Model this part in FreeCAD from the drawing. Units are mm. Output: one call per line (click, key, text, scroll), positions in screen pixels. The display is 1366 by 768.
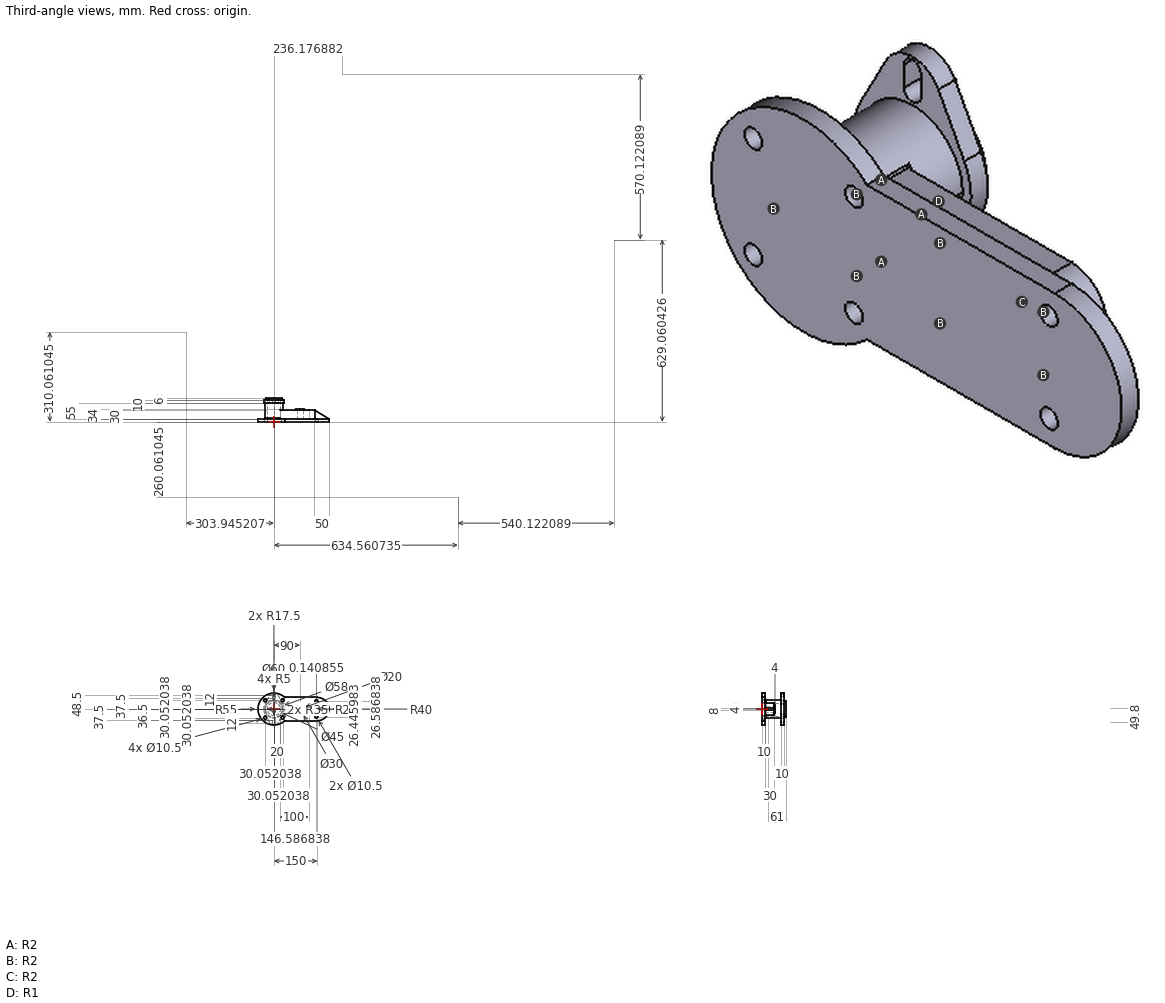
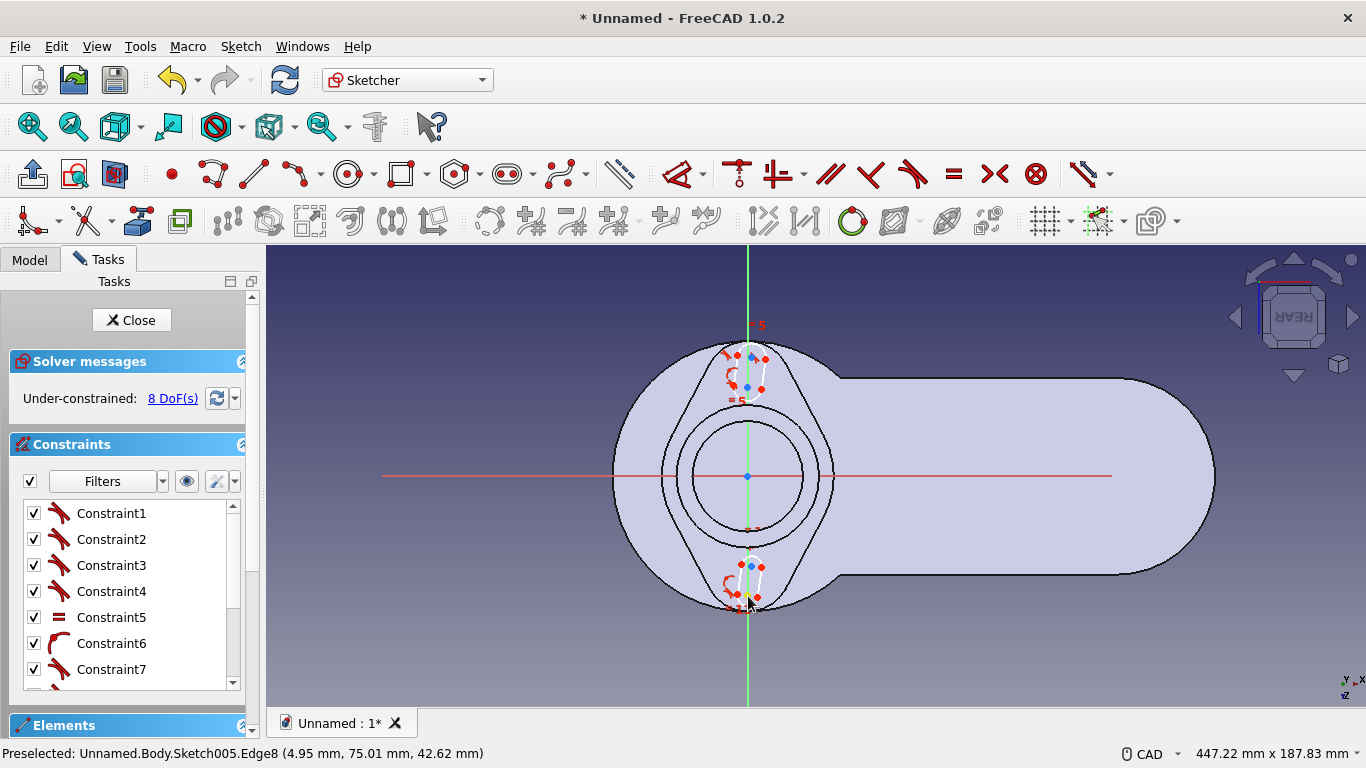
scroll(735, 376, up, 3)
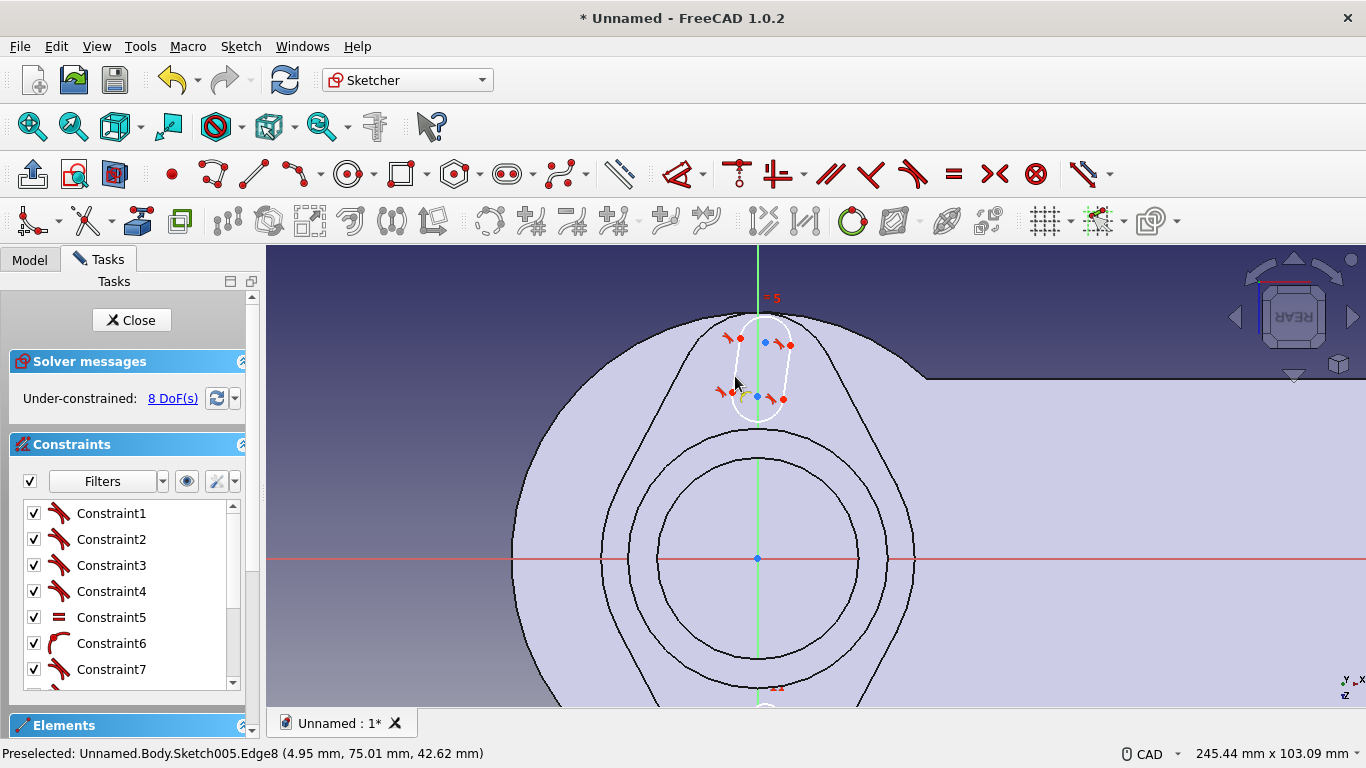
click(735, 376)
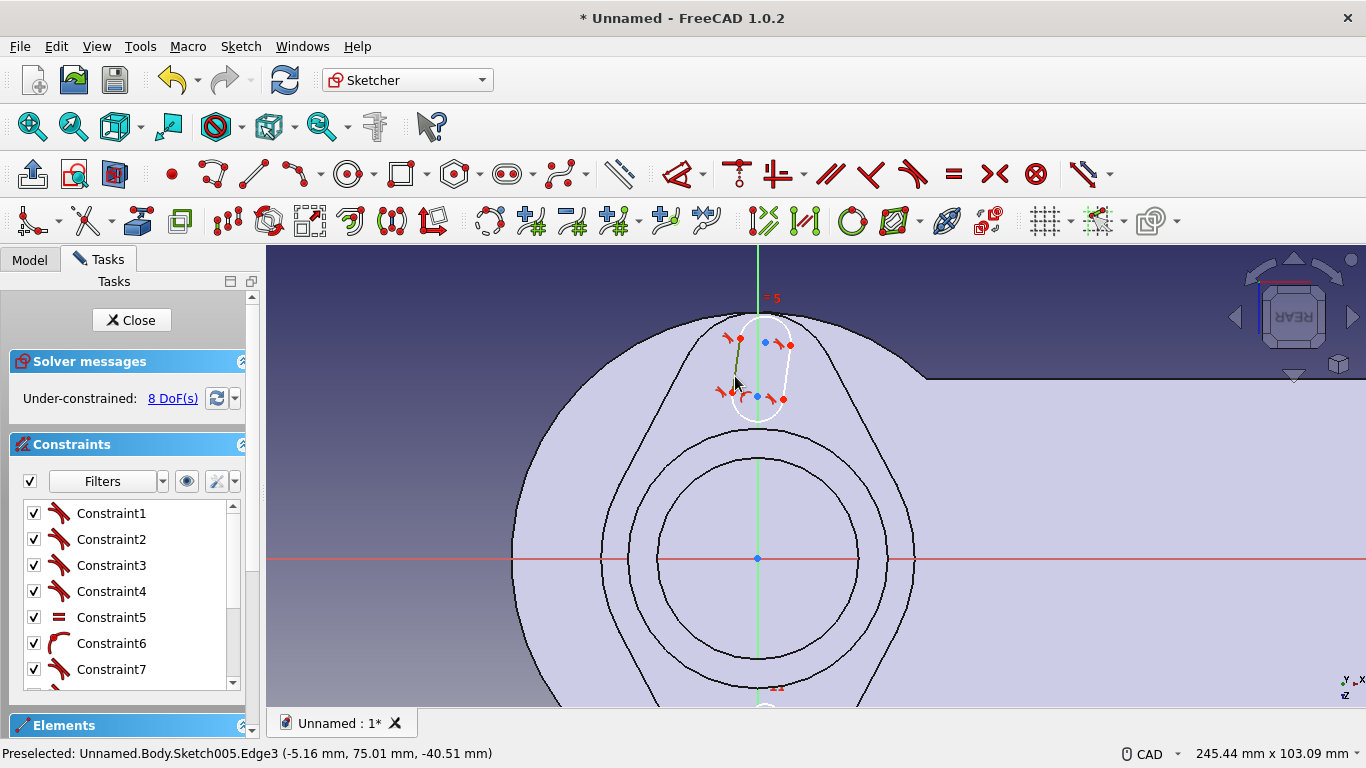
key(v)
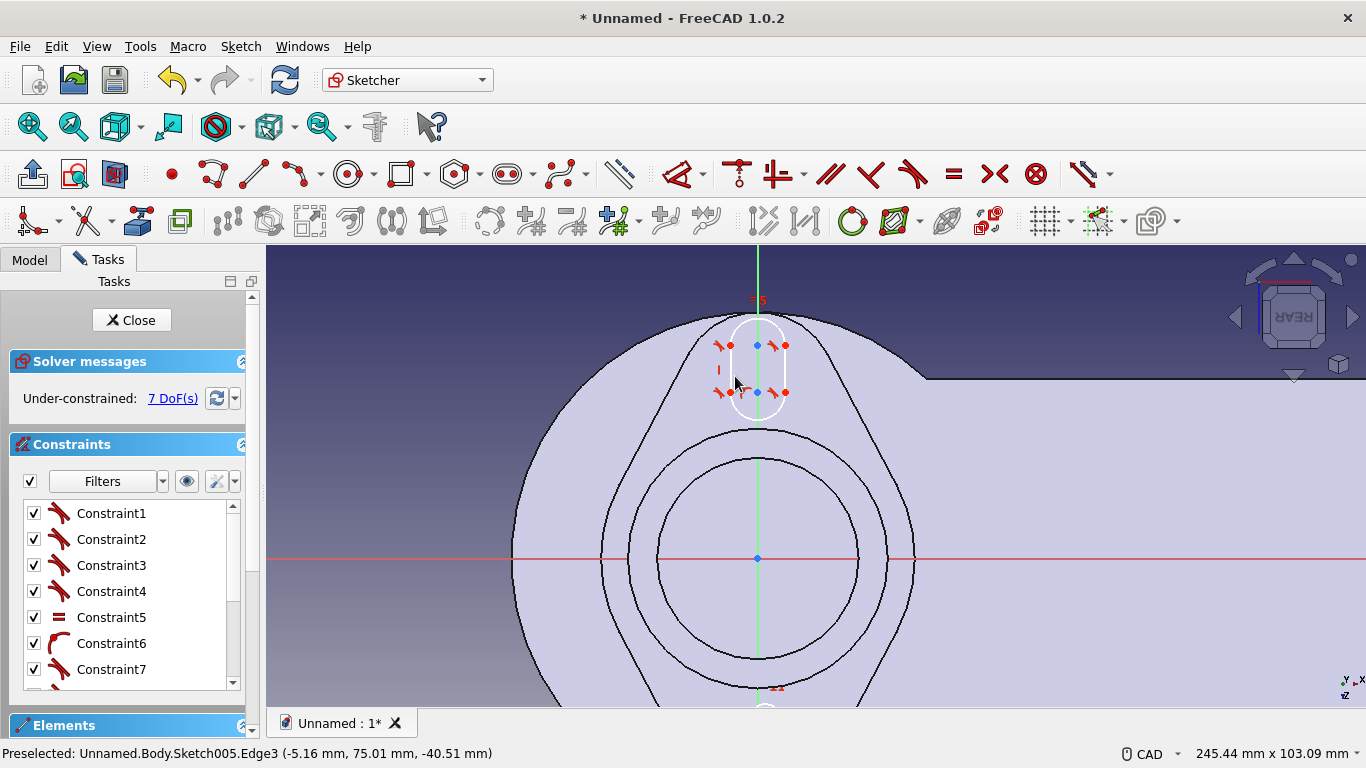
scroll(735, 376, down, 3)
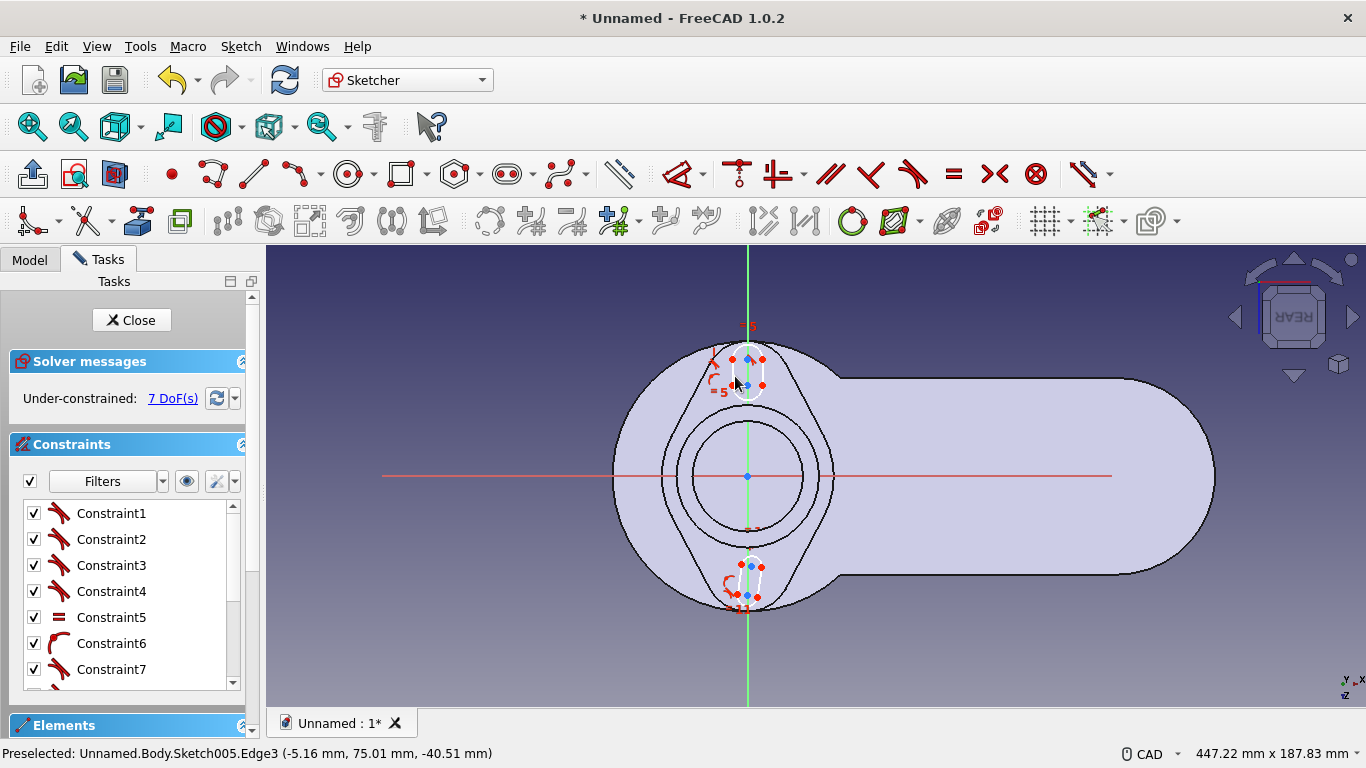
scroll(739, 586, up, 3)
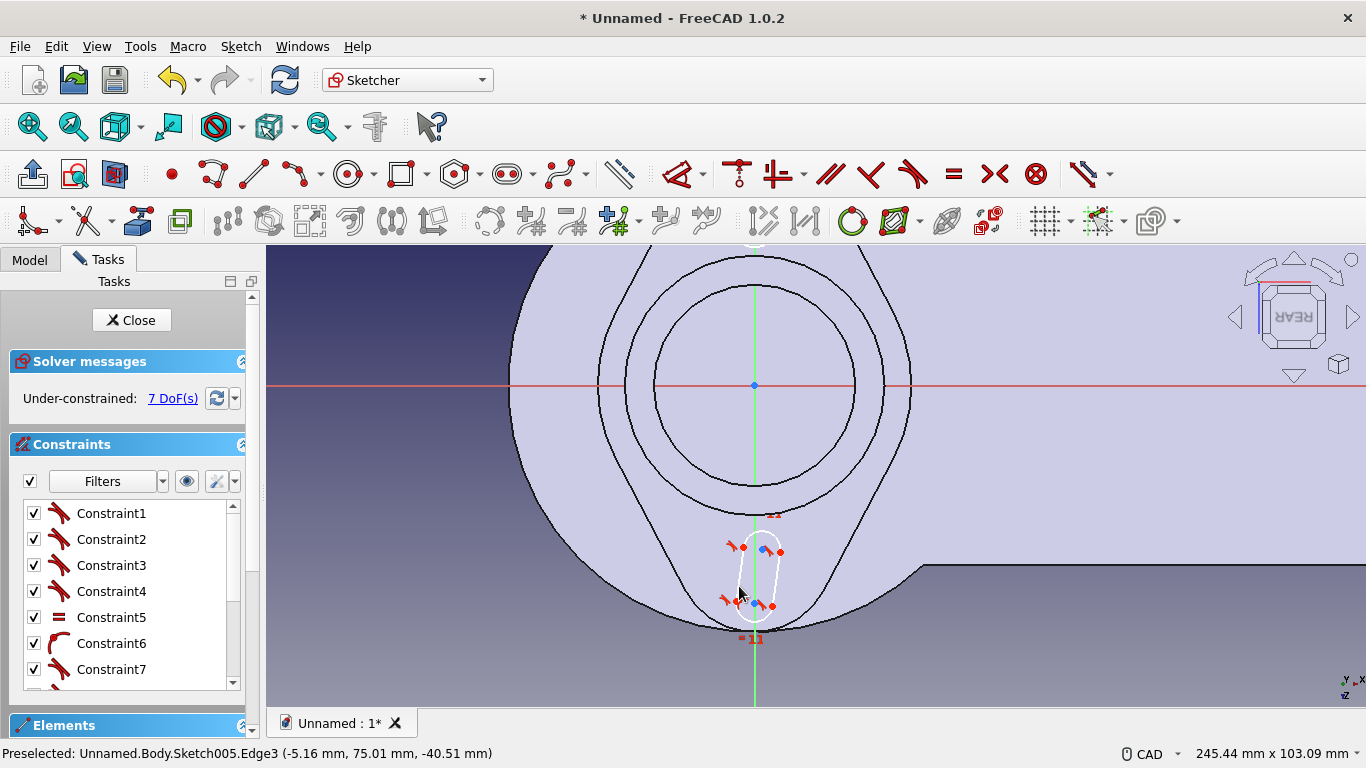
click(739, 585)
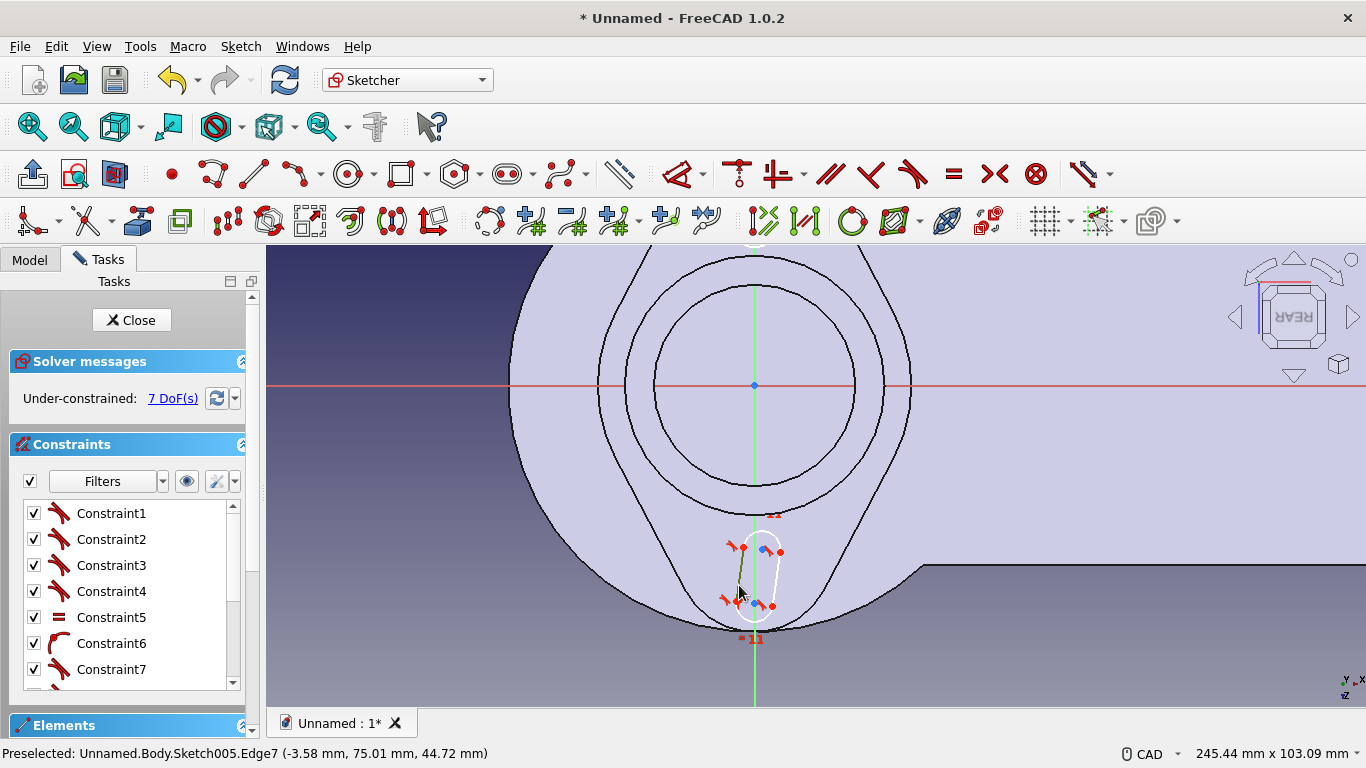
key(v)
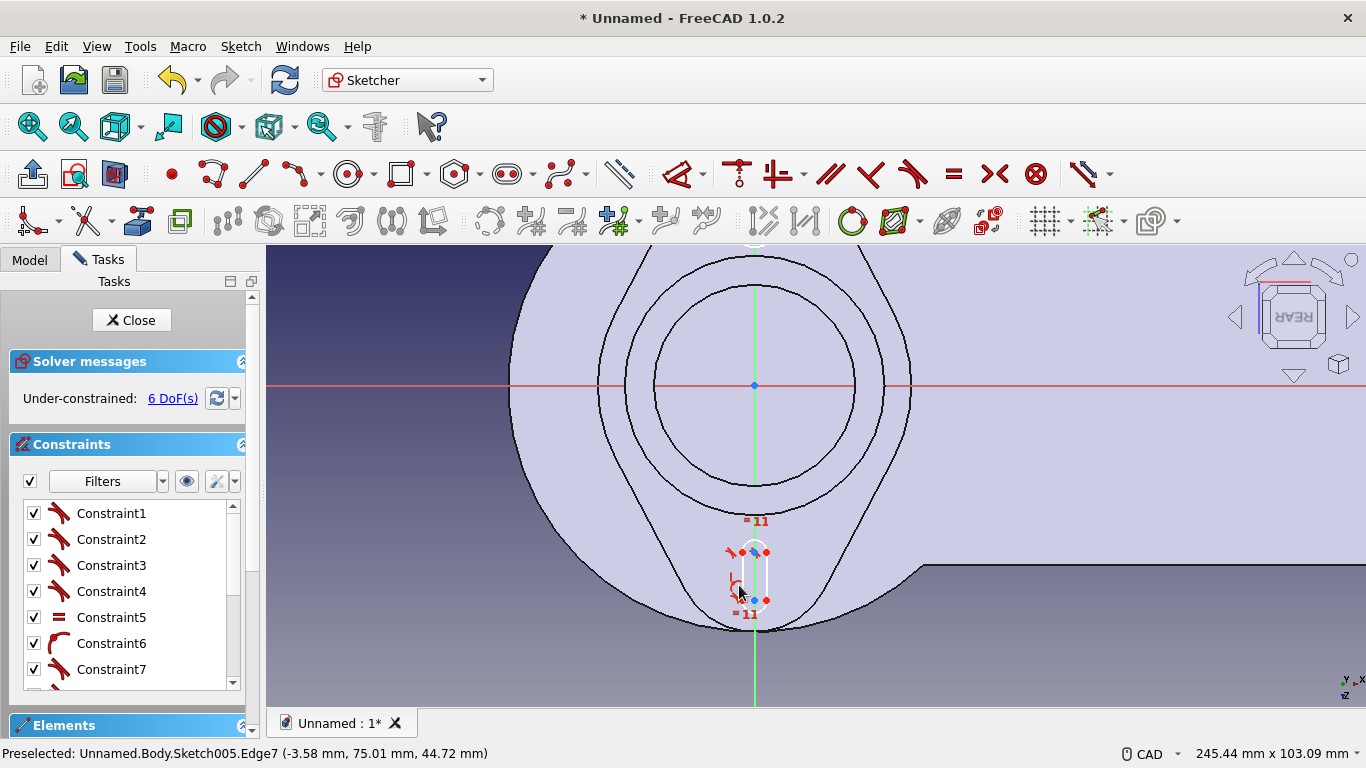
scroll(739, 586, down, 3)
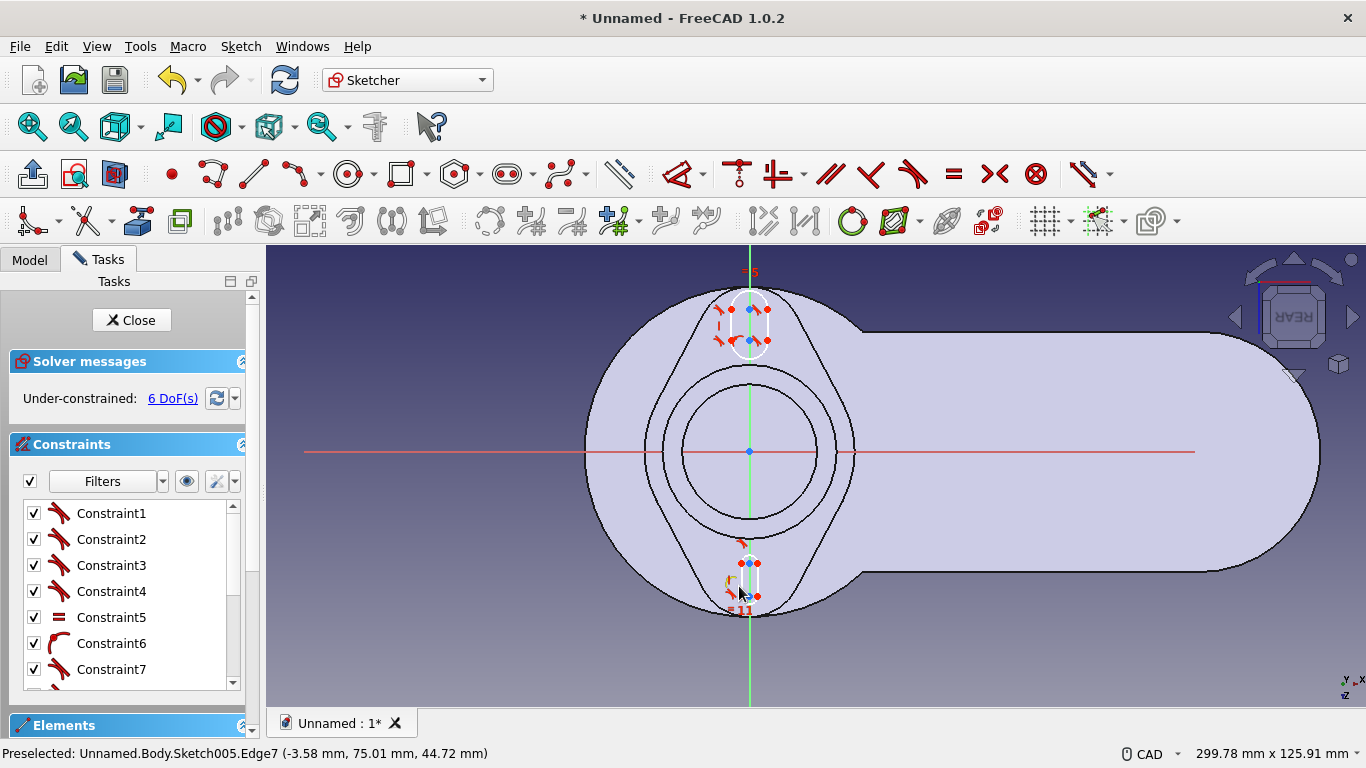
scroll(739, 397, up, 3)